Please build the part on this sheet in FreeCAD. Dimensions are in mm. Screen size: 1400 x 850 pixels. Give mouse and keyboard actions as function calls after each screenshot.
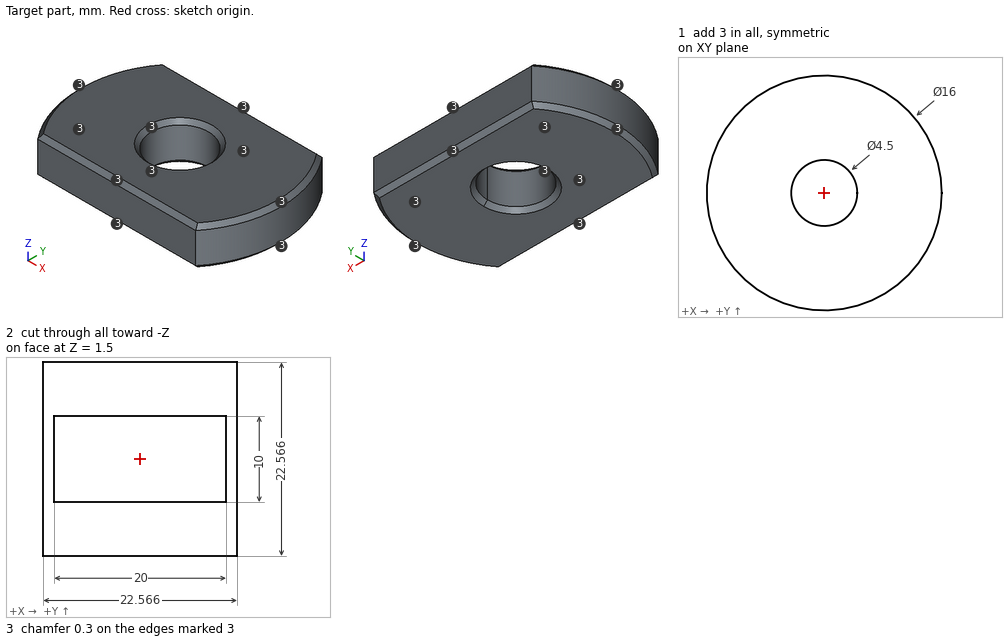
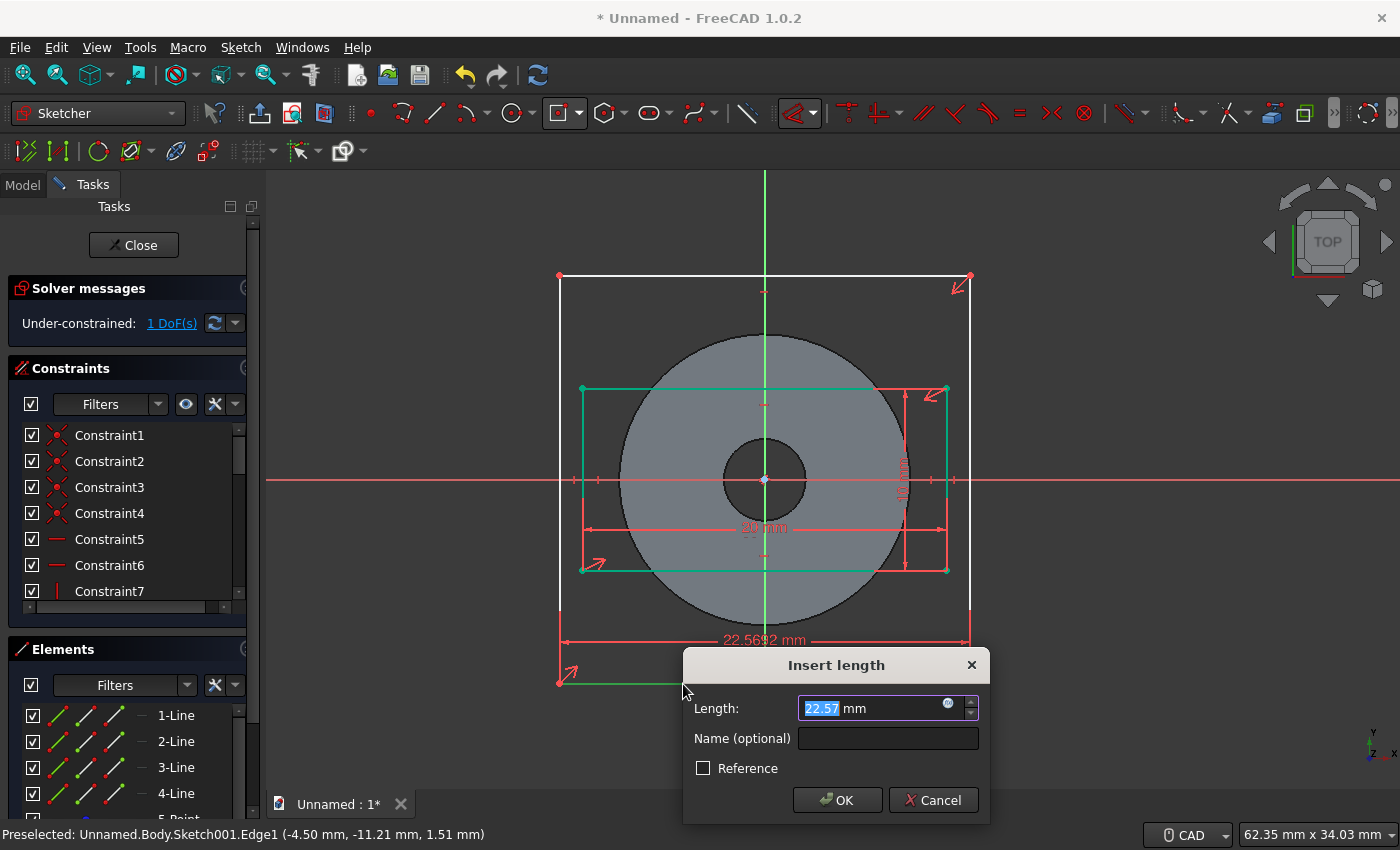
text(22.566)
key(Return)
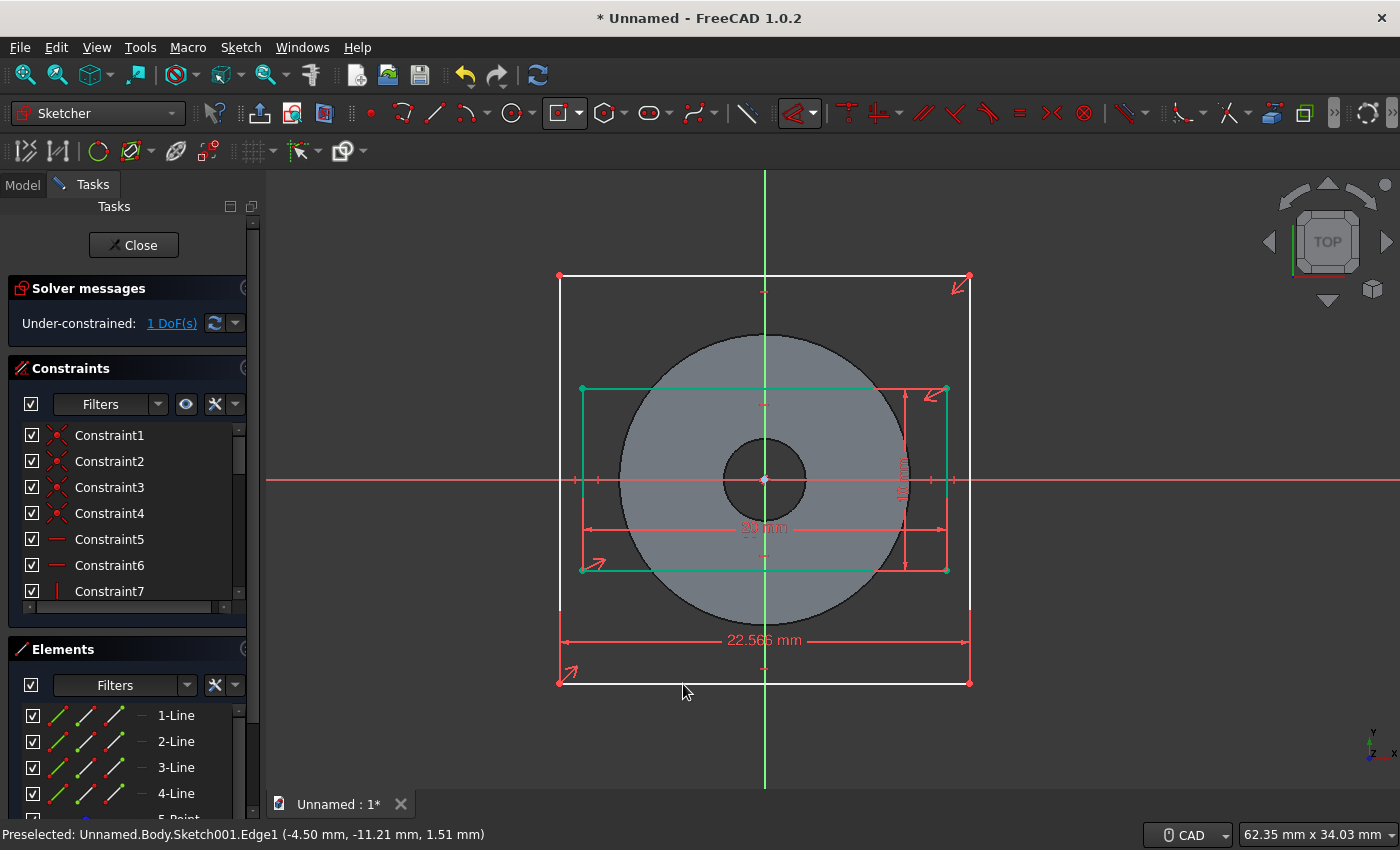
click(970, 561)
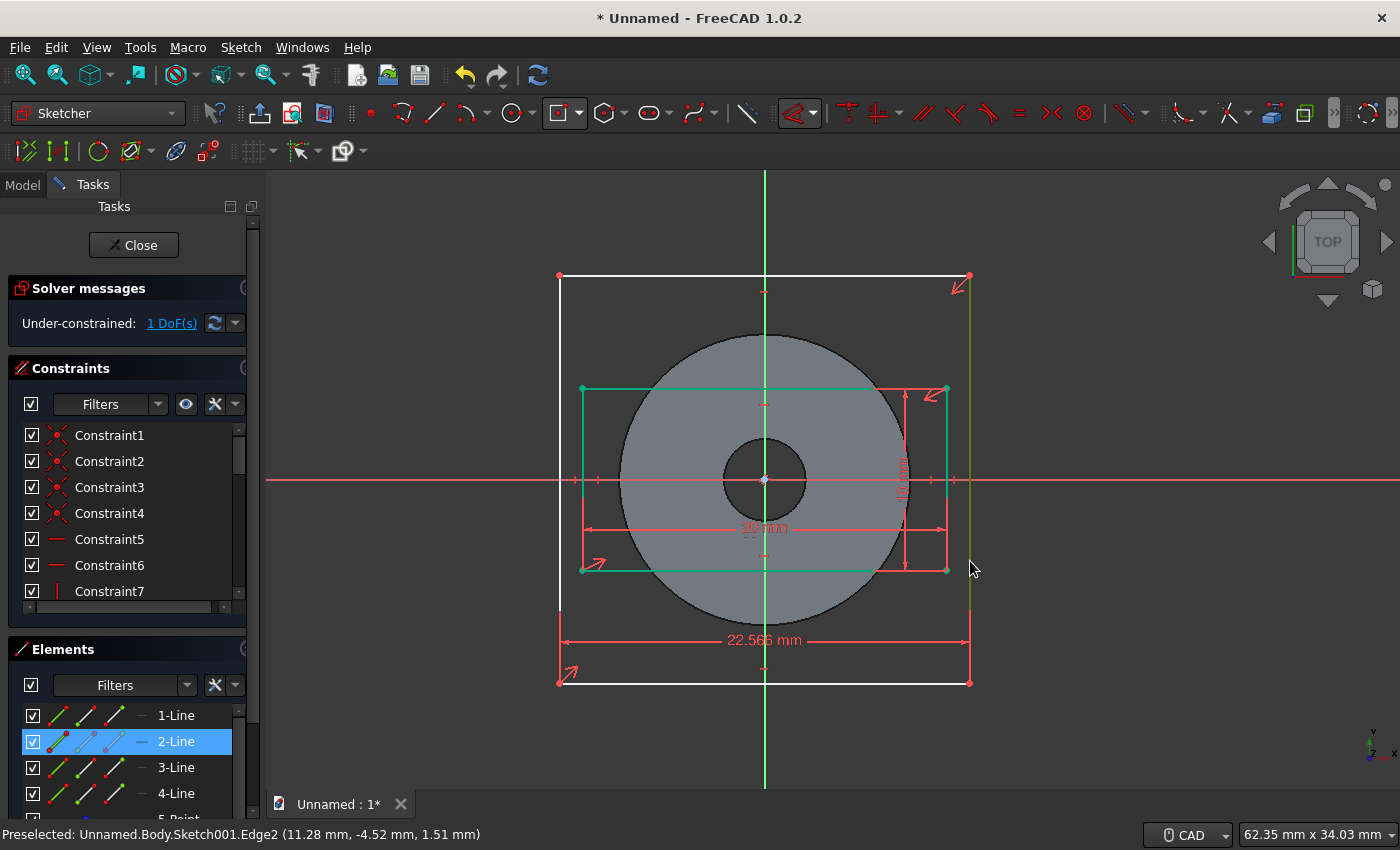
key(i)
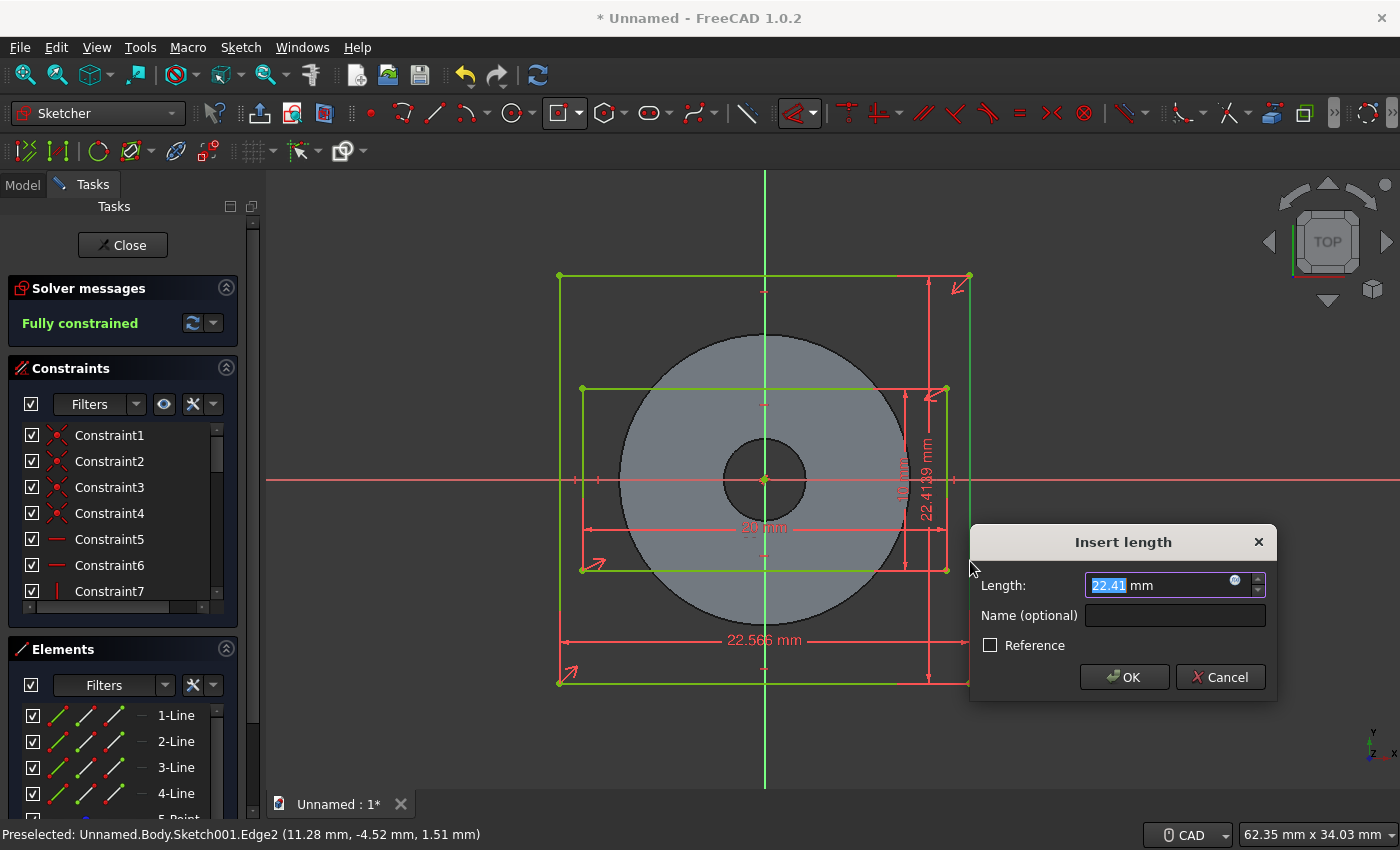
text(22.566)
key(Return)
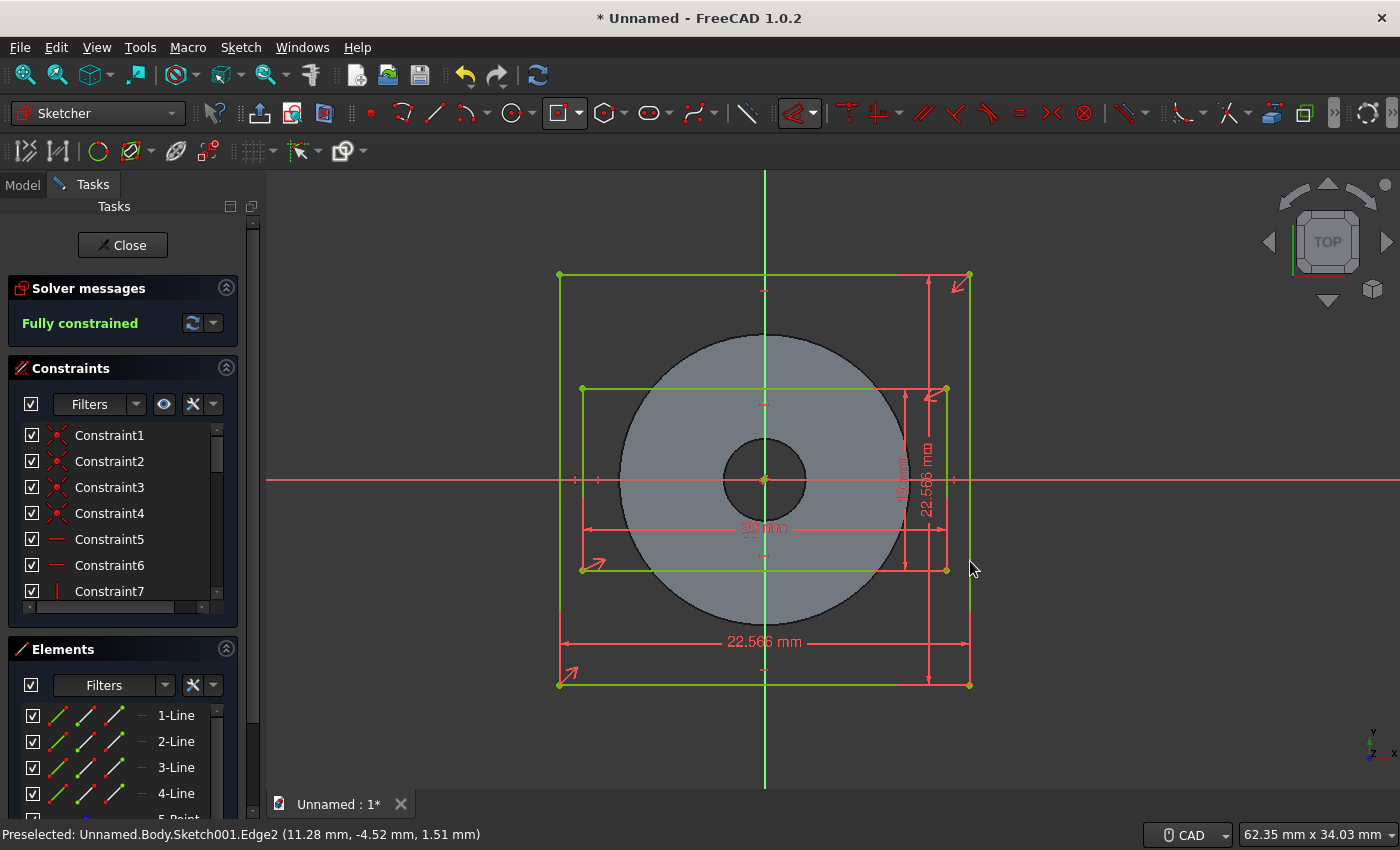
click(123, 245)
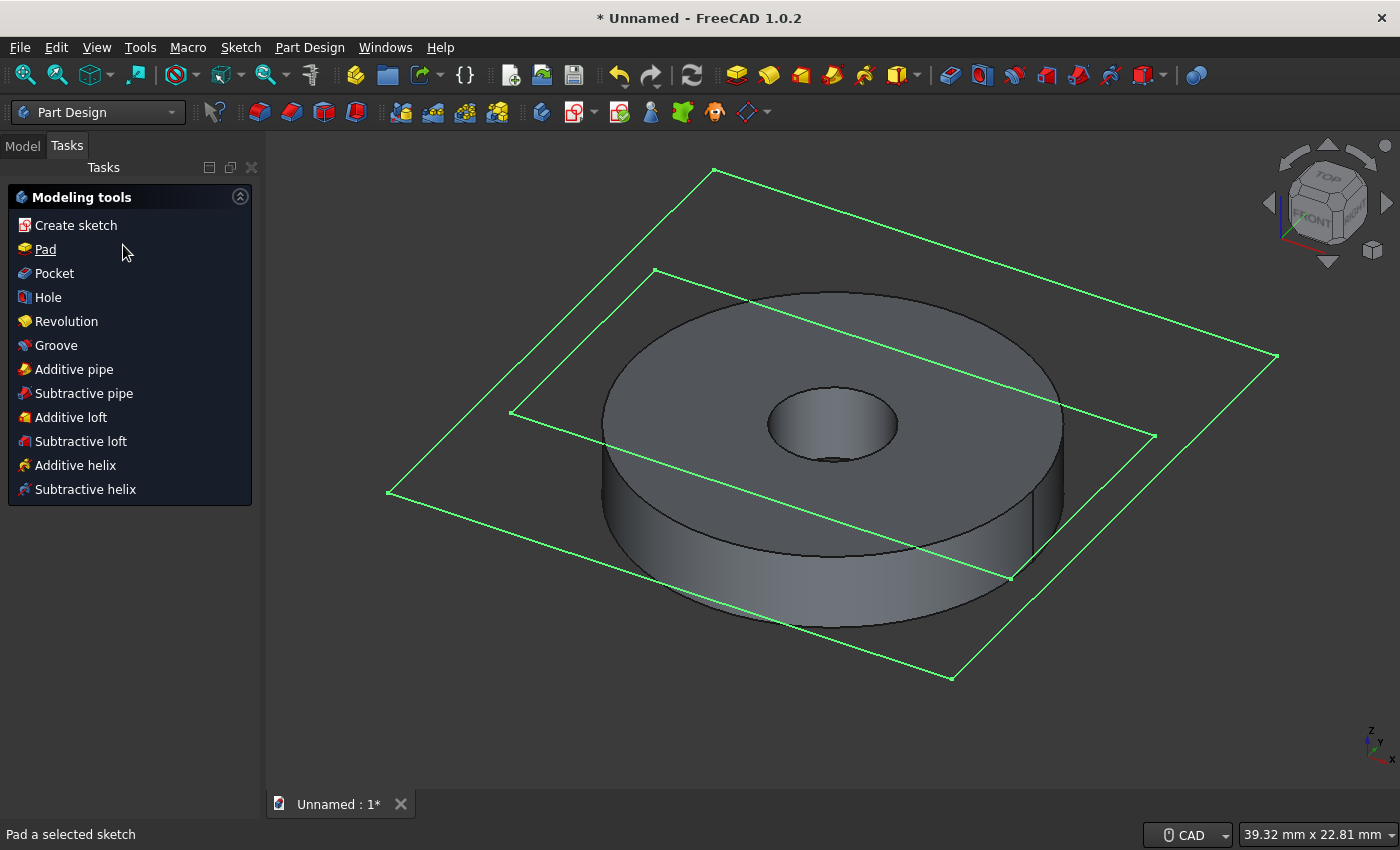
click(952, 76)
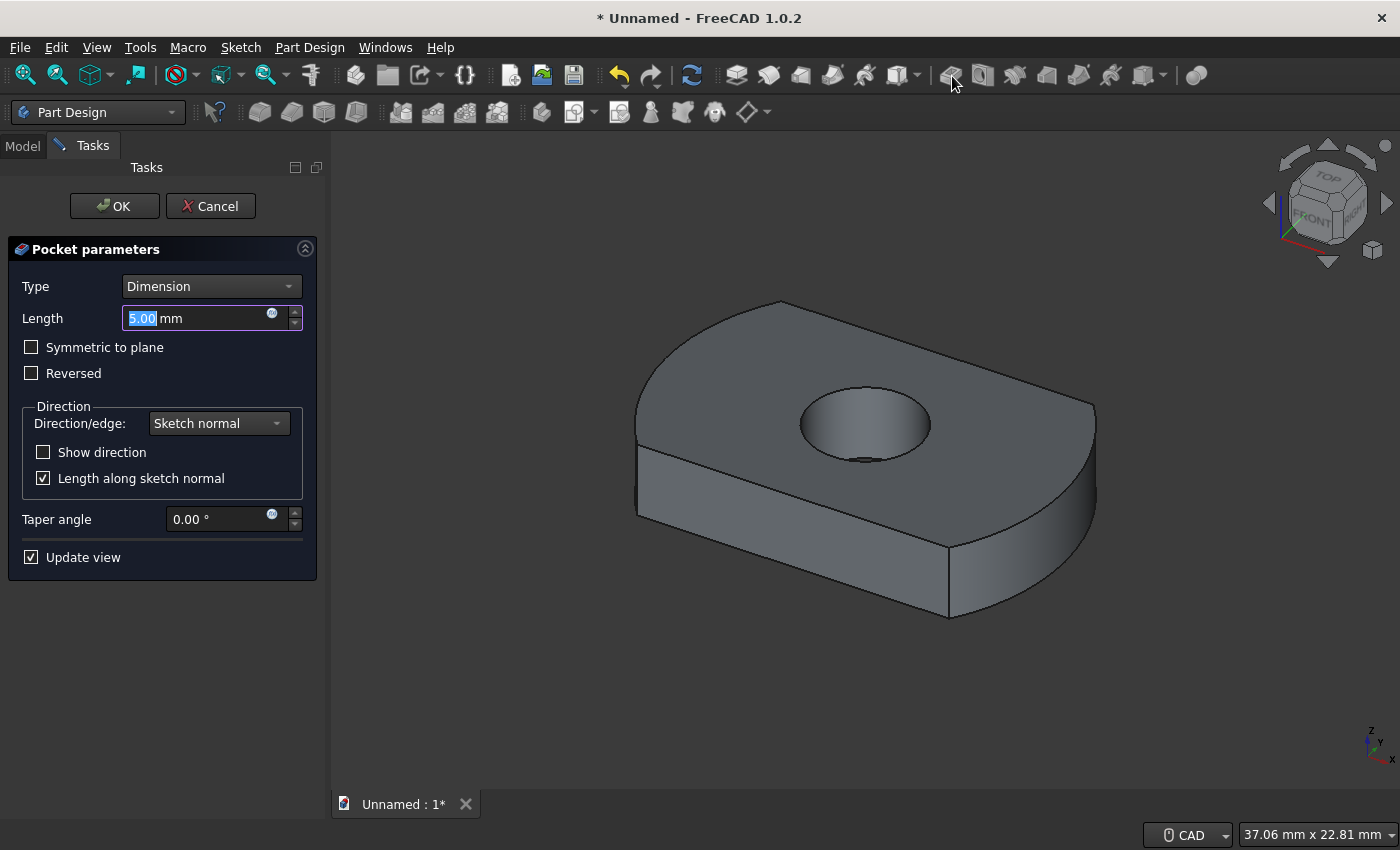
click(212, 286)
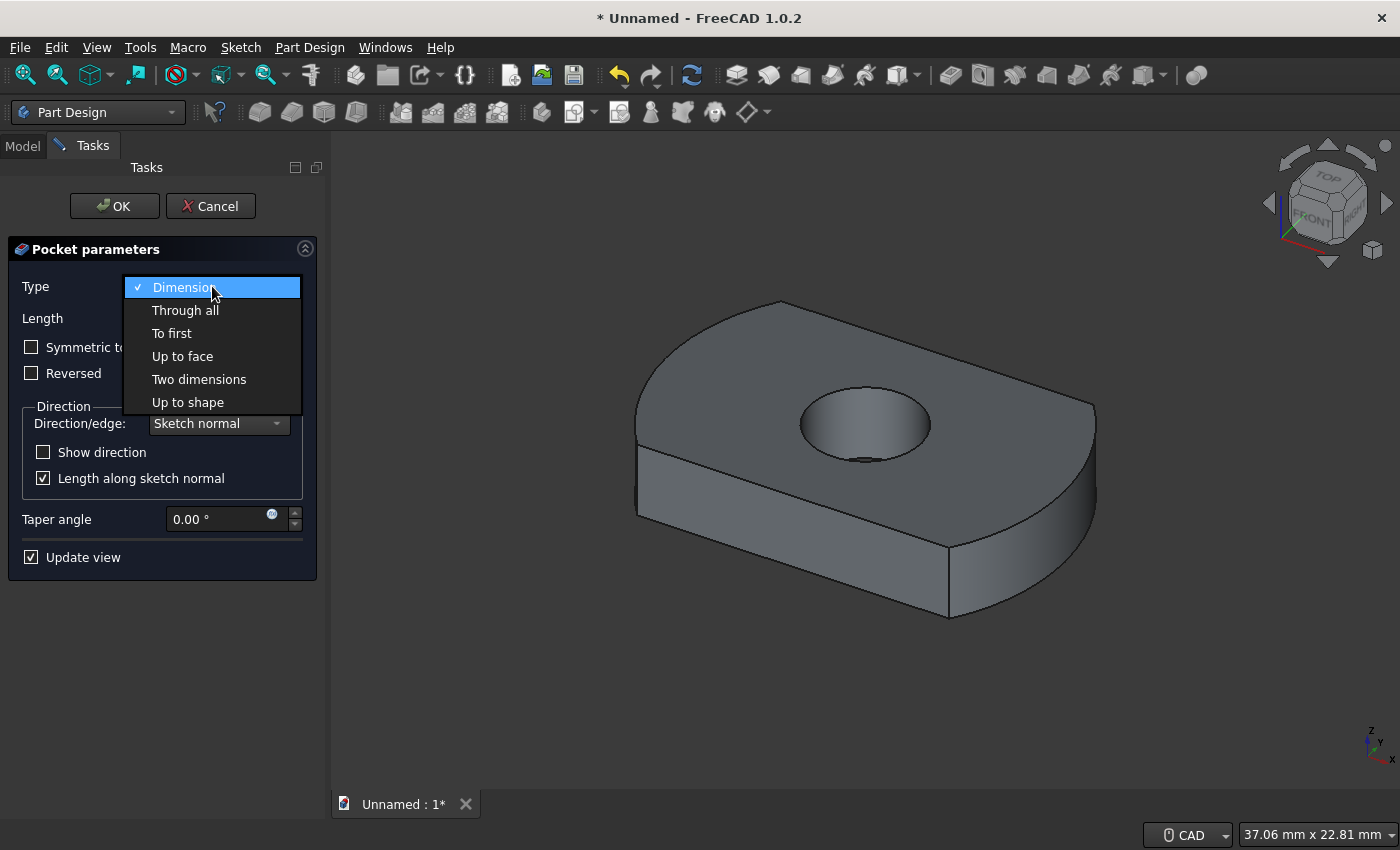
click(212, 310)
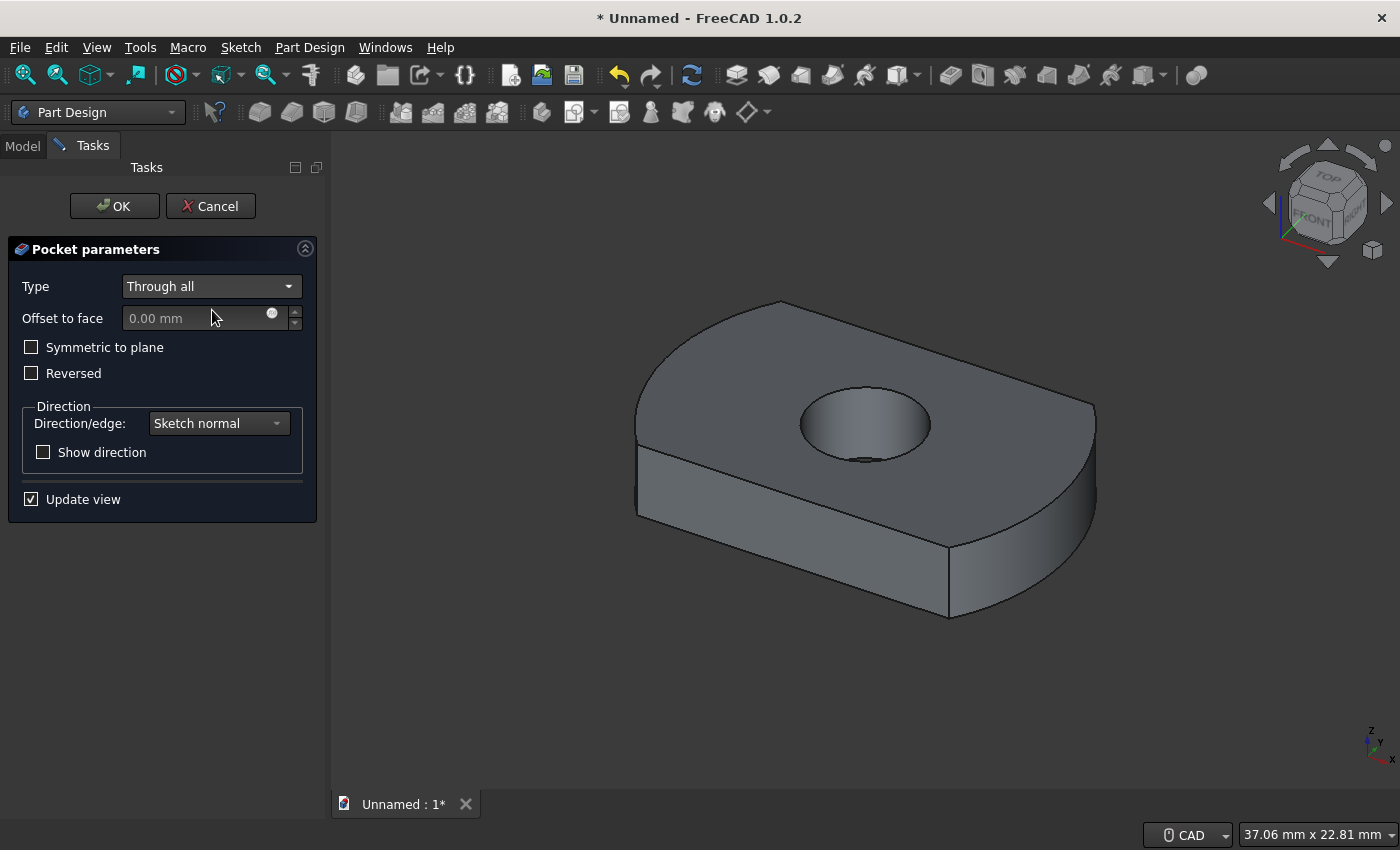
click(115, 206)